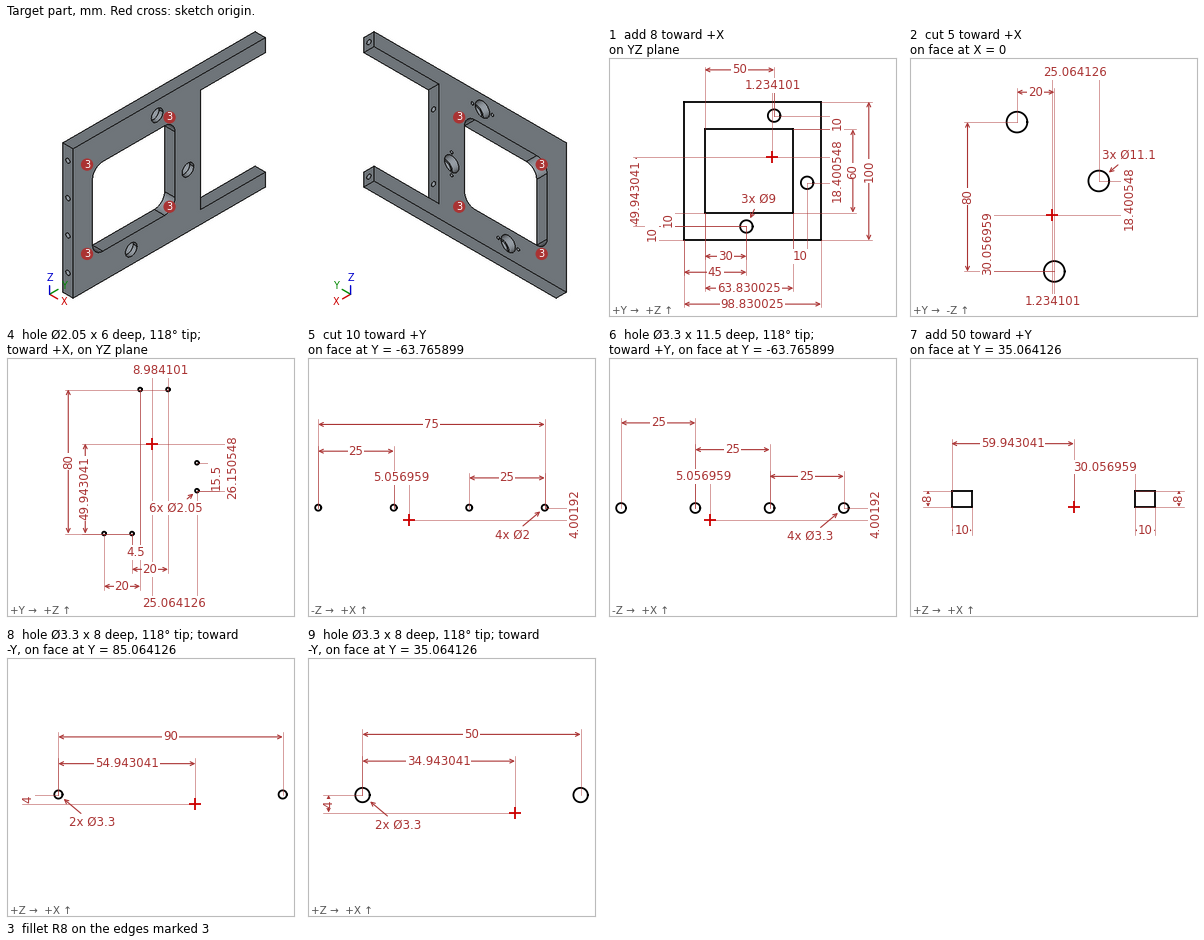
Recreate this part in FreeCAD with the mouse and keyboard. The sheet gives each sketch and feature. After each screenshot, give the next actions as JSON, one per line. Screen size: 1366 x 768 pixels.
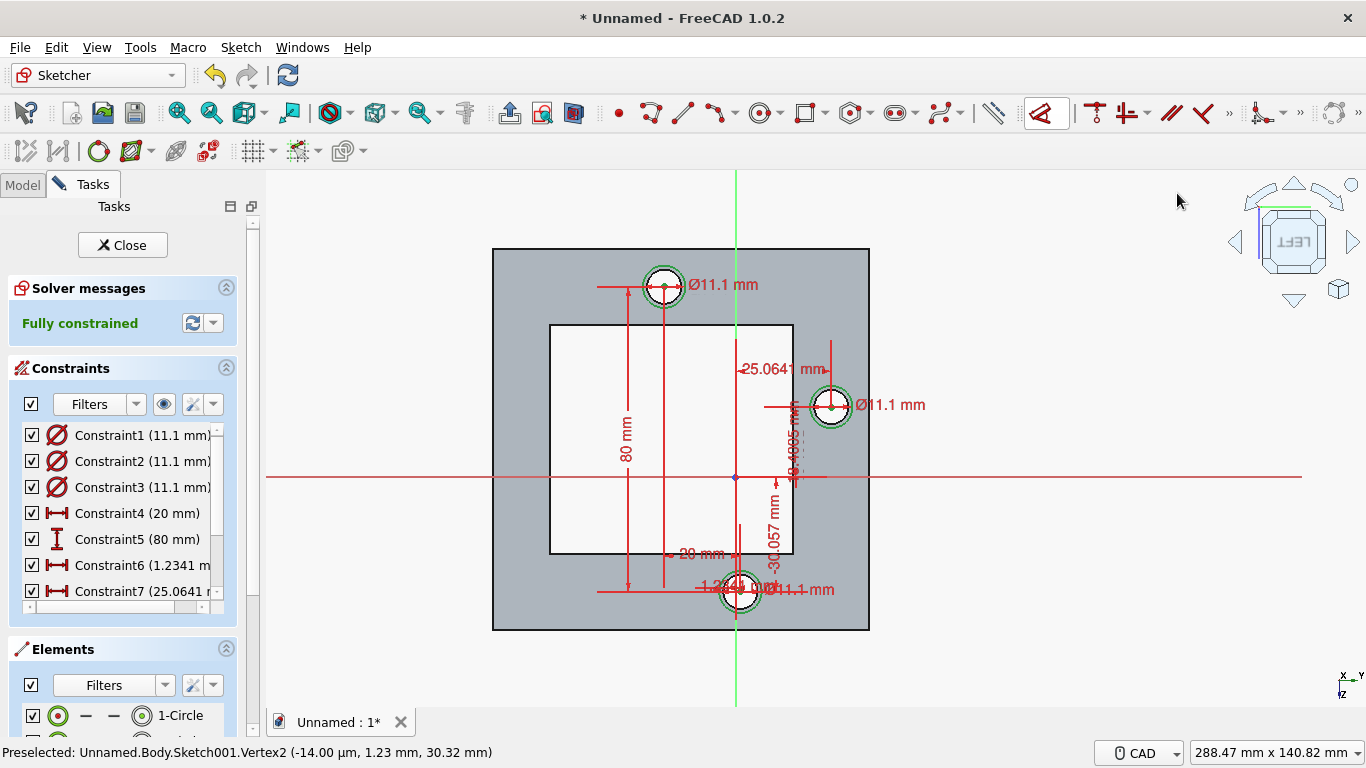
{"action": "left_click", "coordinate": [123, 245]}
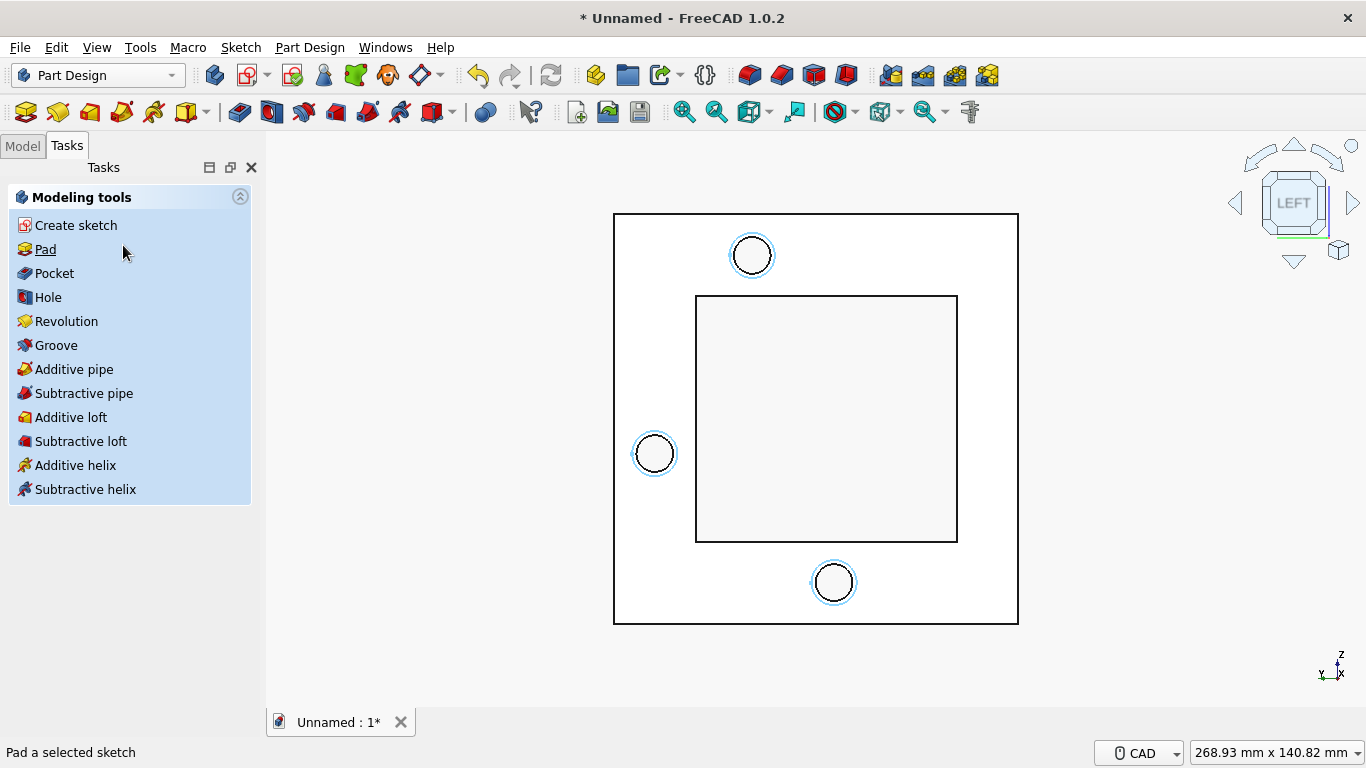
{"action": "left_click", "coordinate": [240, 112]}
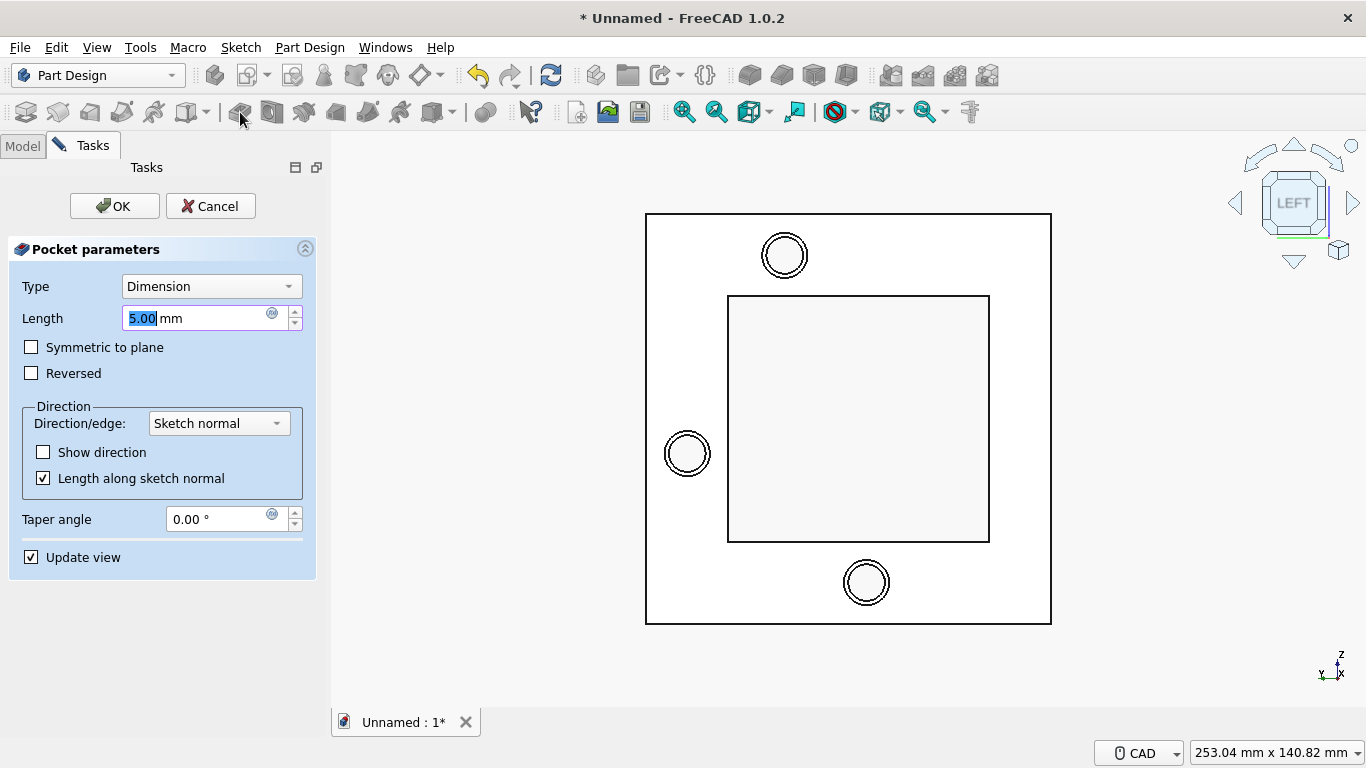
{"action": "type", "text": "5"}
{"action": "key", "text": "Tab"}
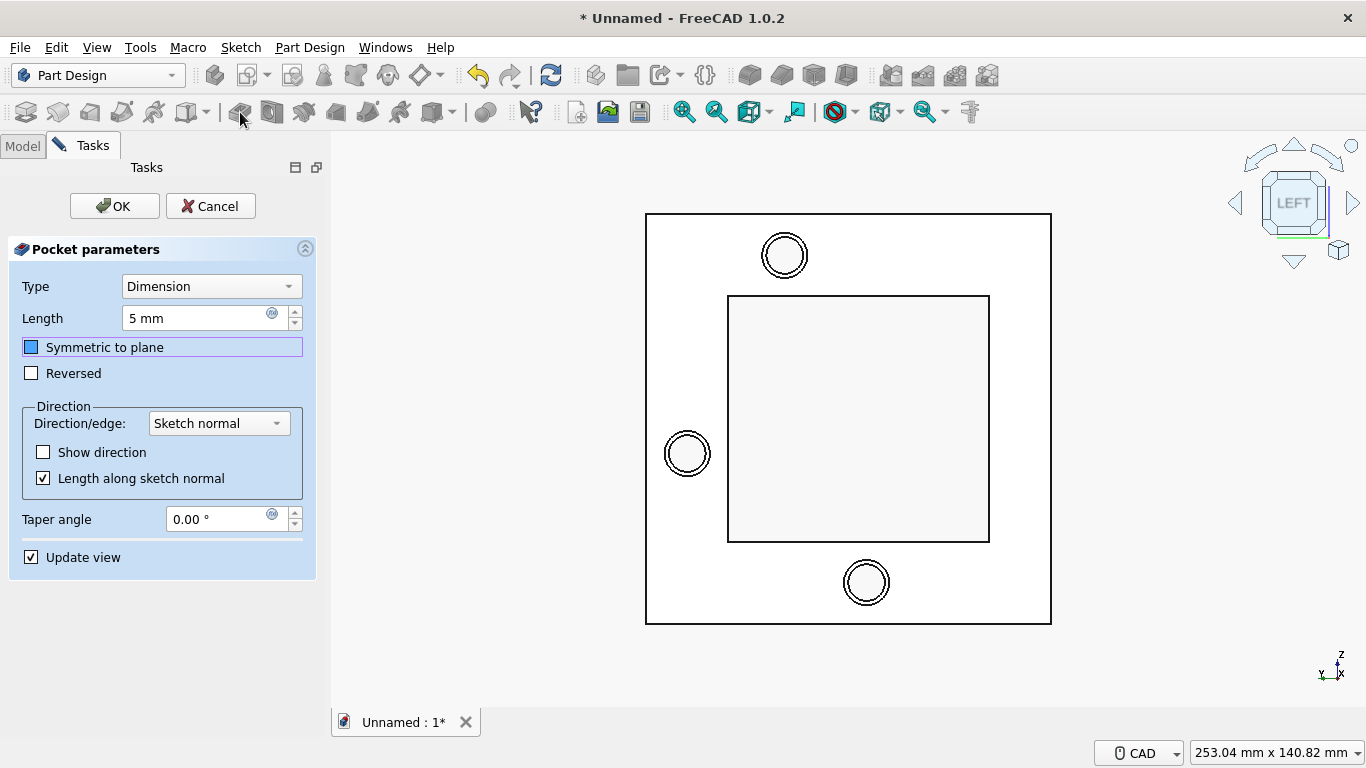
{"action": "left_click", "coordinate": [115, 206]}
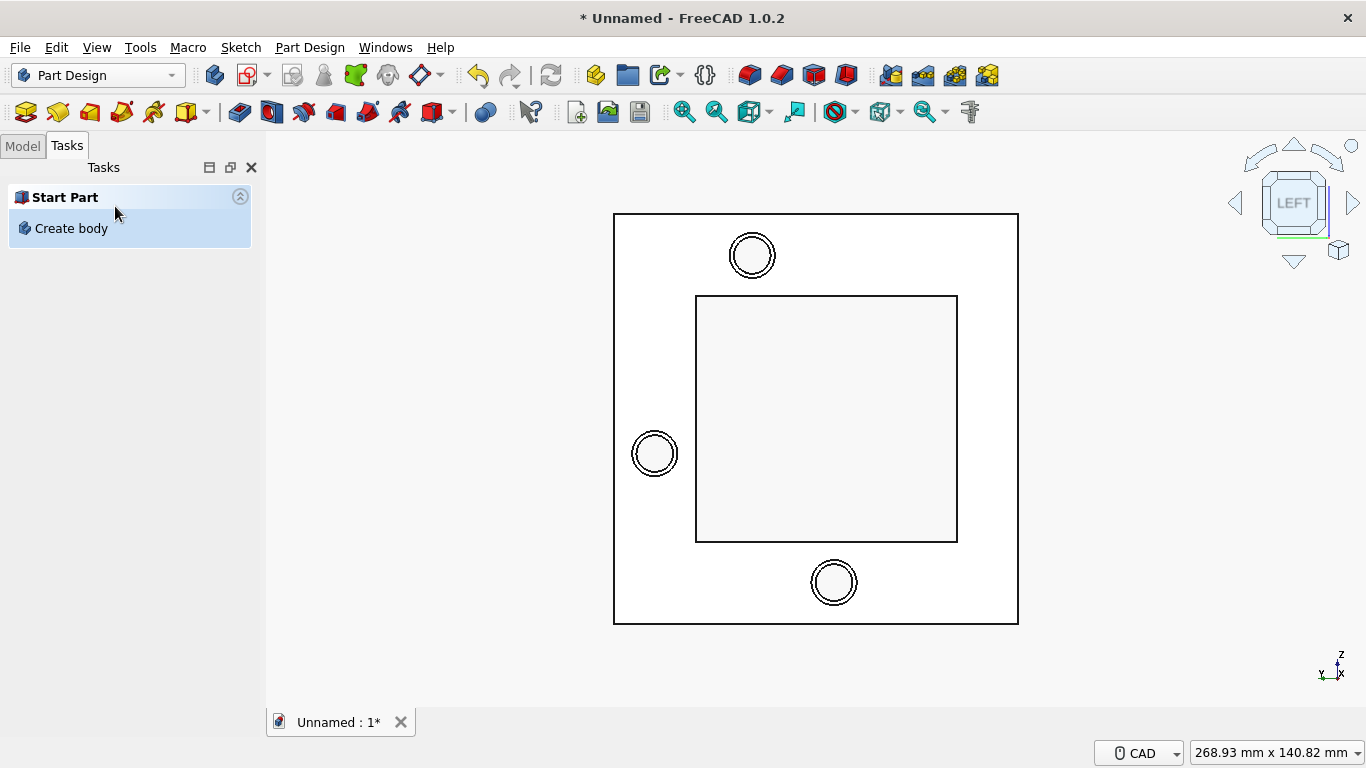
{"action": "key", "text": "0"}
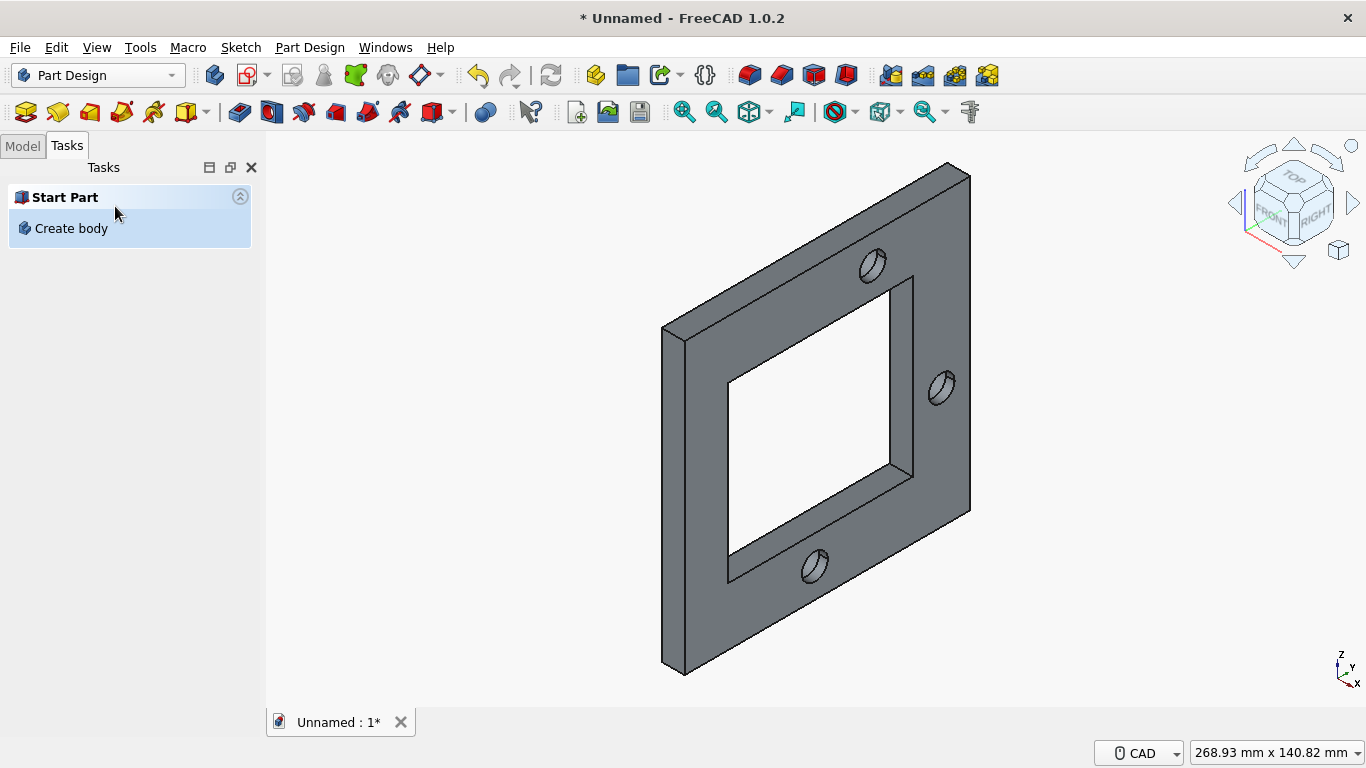
{"action": "key", "text": "2"}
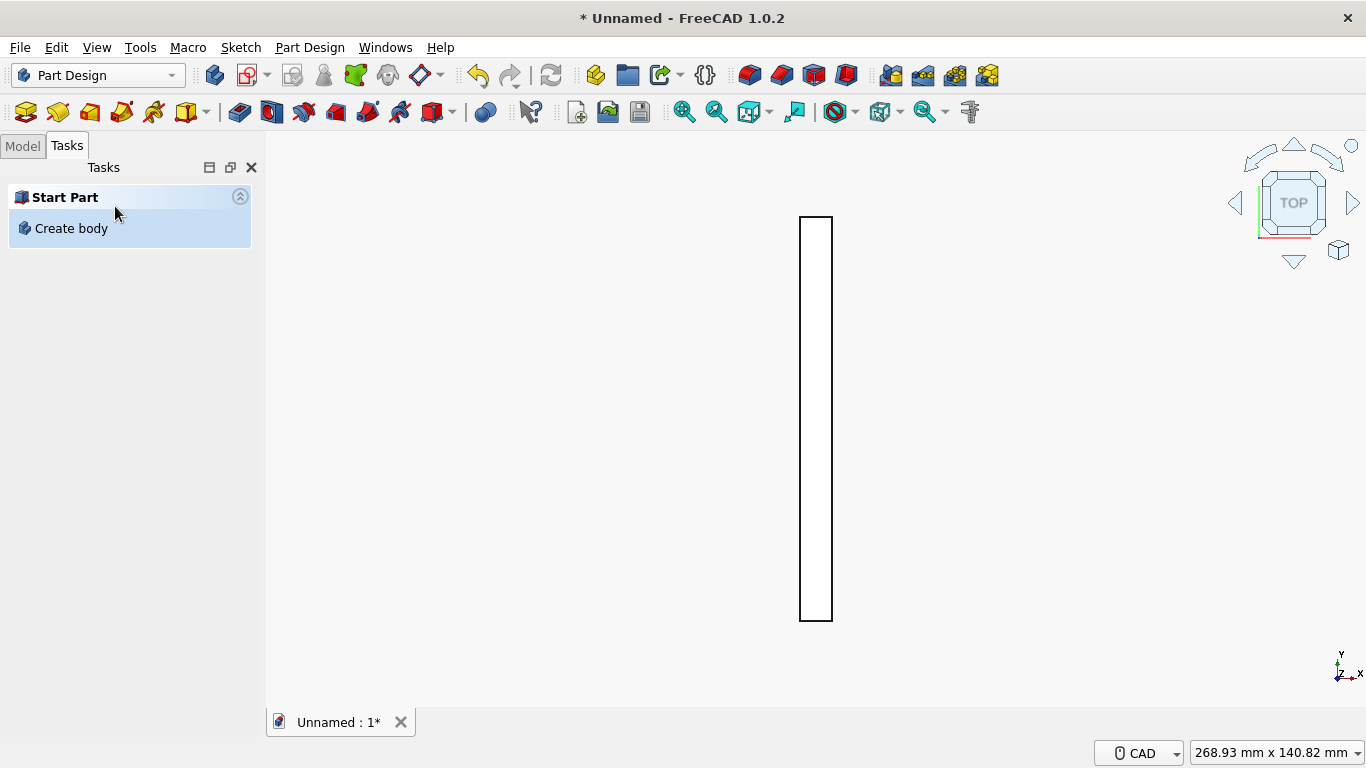
{"action": "key", "text": "1"}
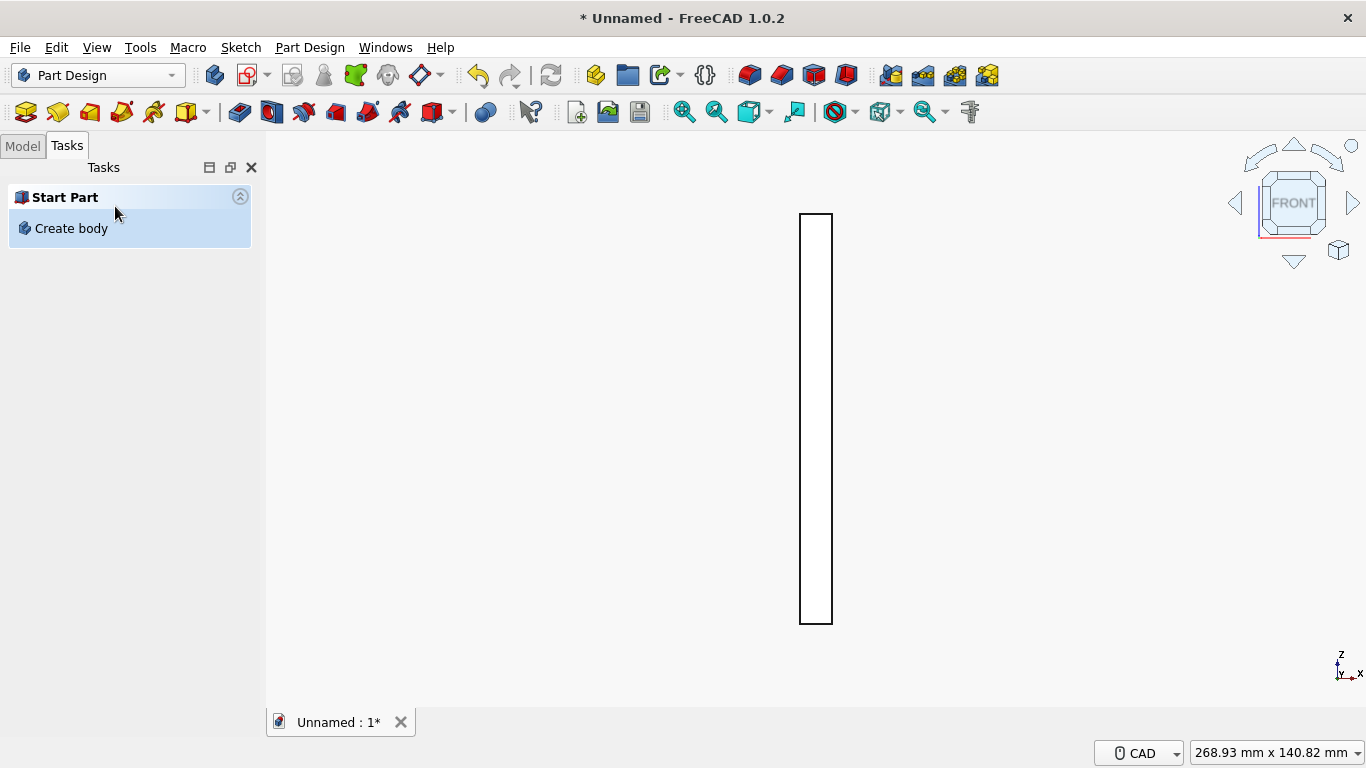
{"action": "key", "text": "3"}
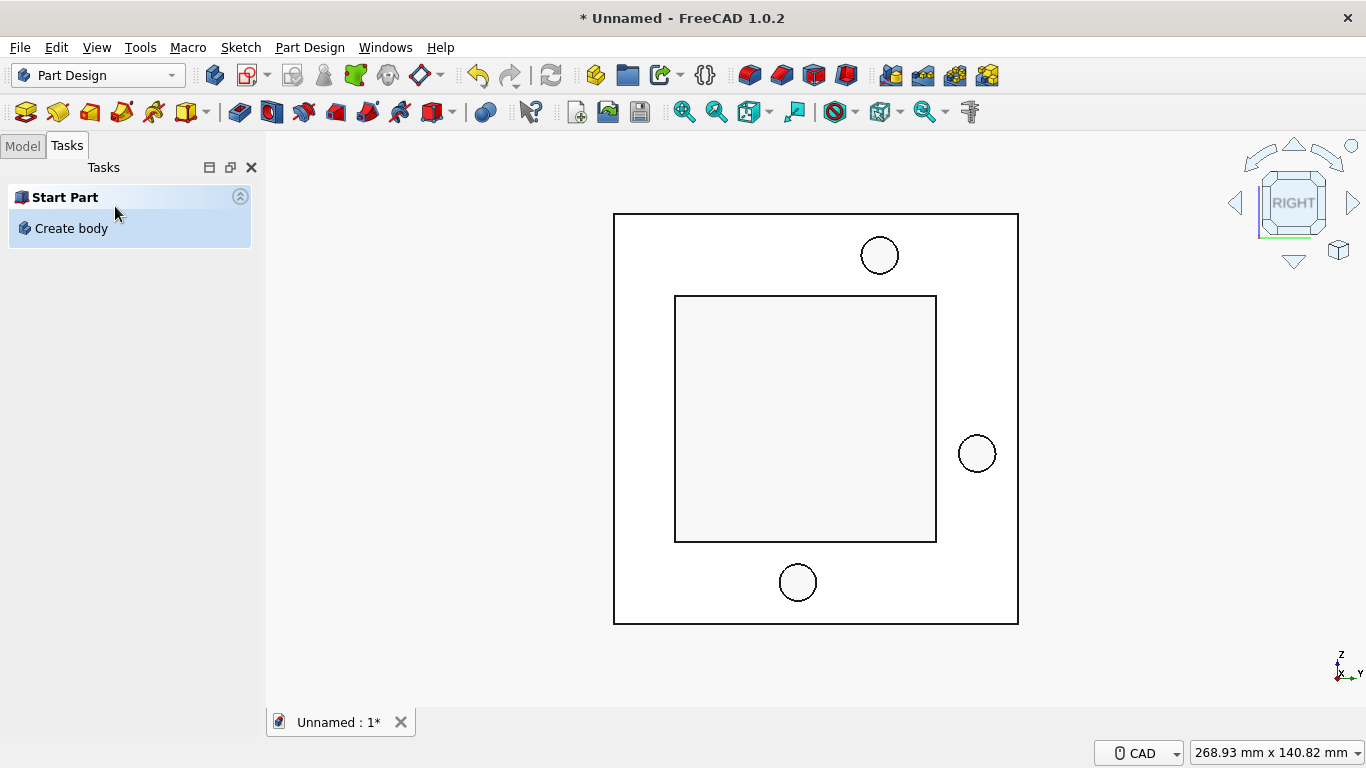
{"action": "key", "text": "5"}